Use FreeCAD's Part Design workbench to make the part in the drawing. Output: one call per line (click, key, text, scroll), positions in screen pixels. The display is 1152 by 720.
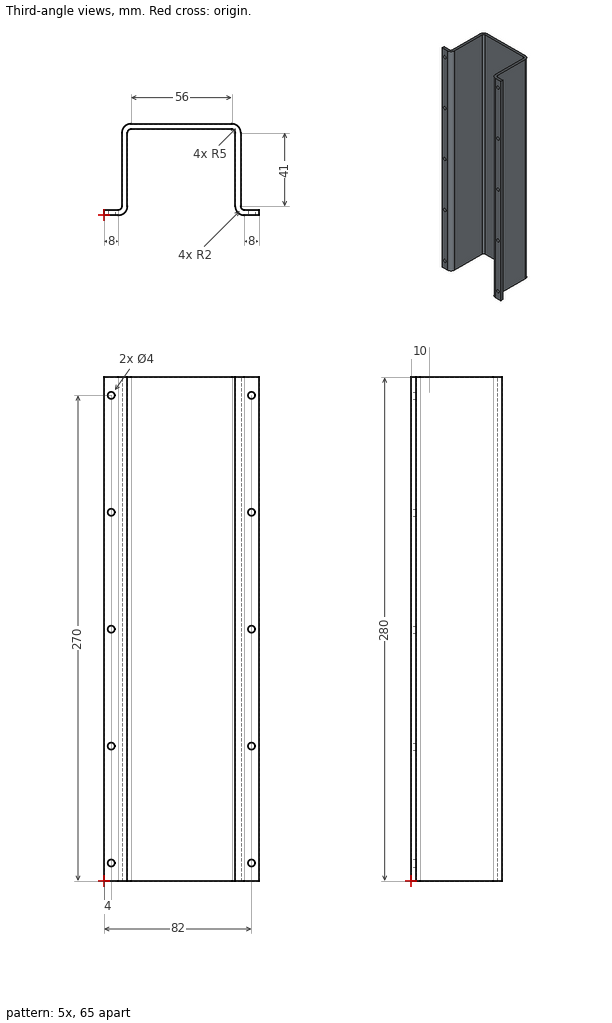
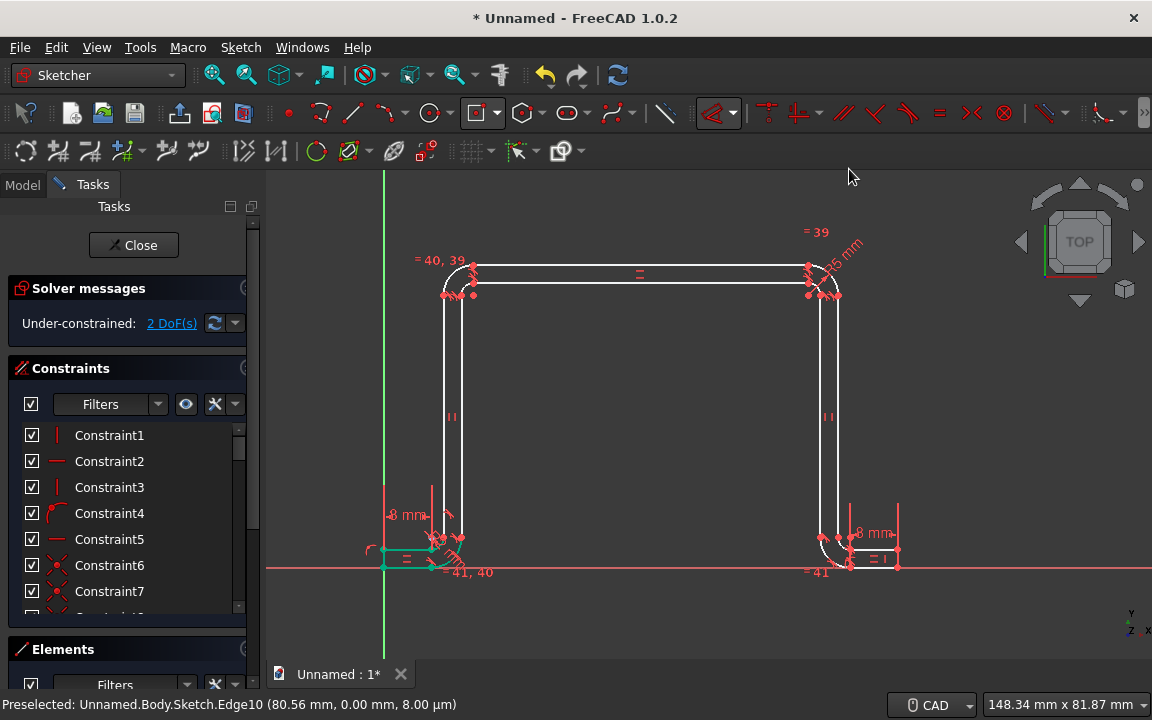
click(838, 465)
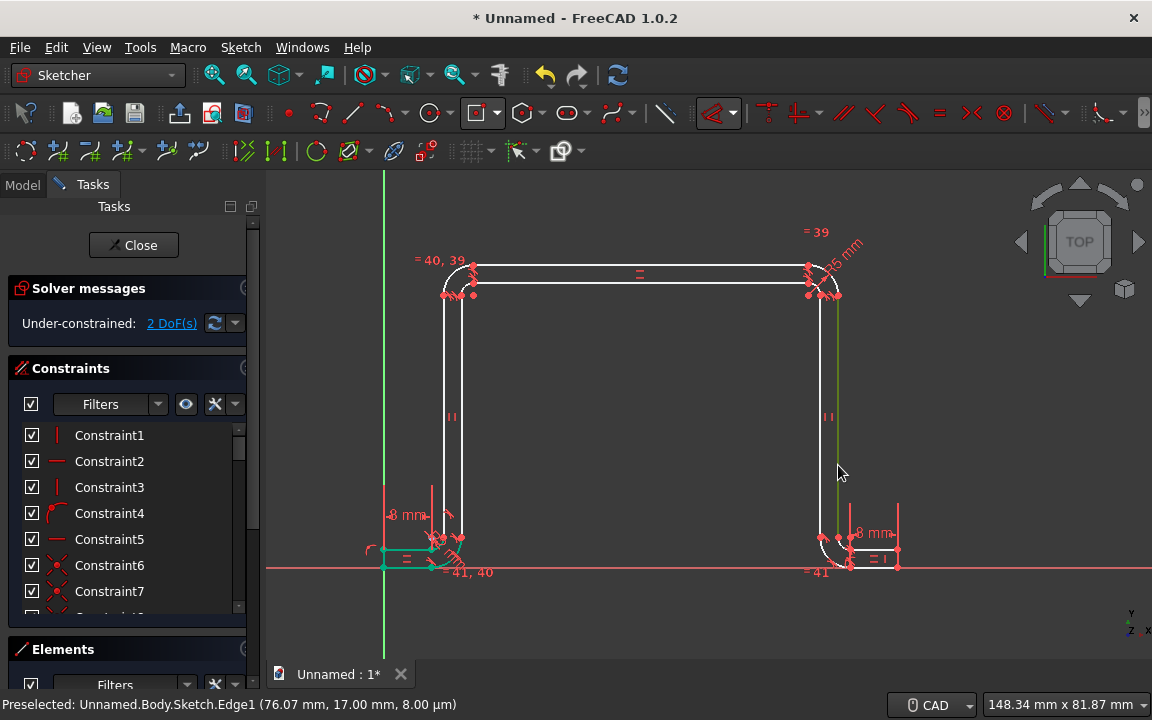
key(i)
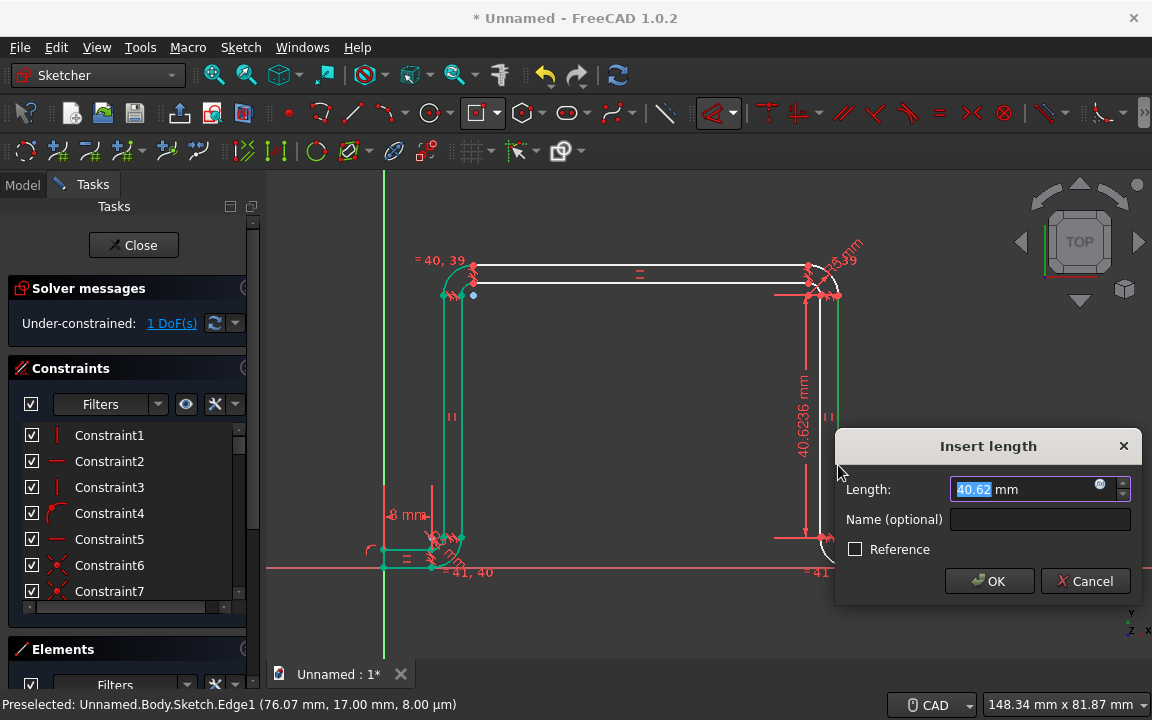
text(41)
key(Return)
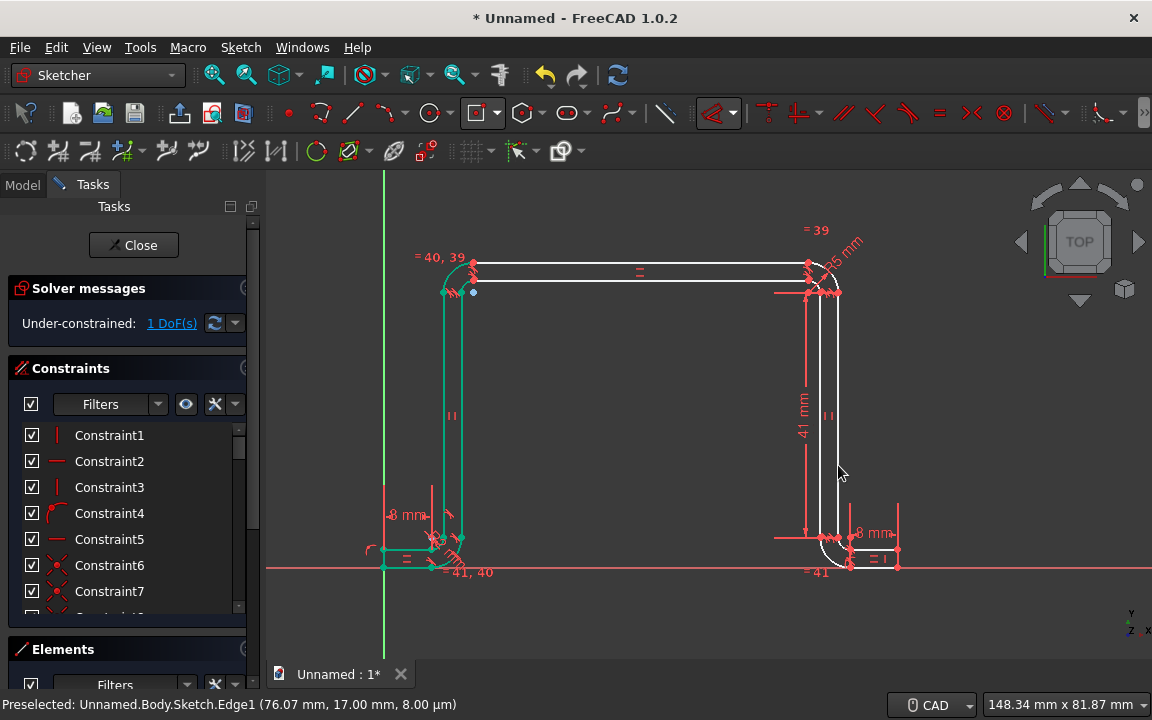
click(708, 263)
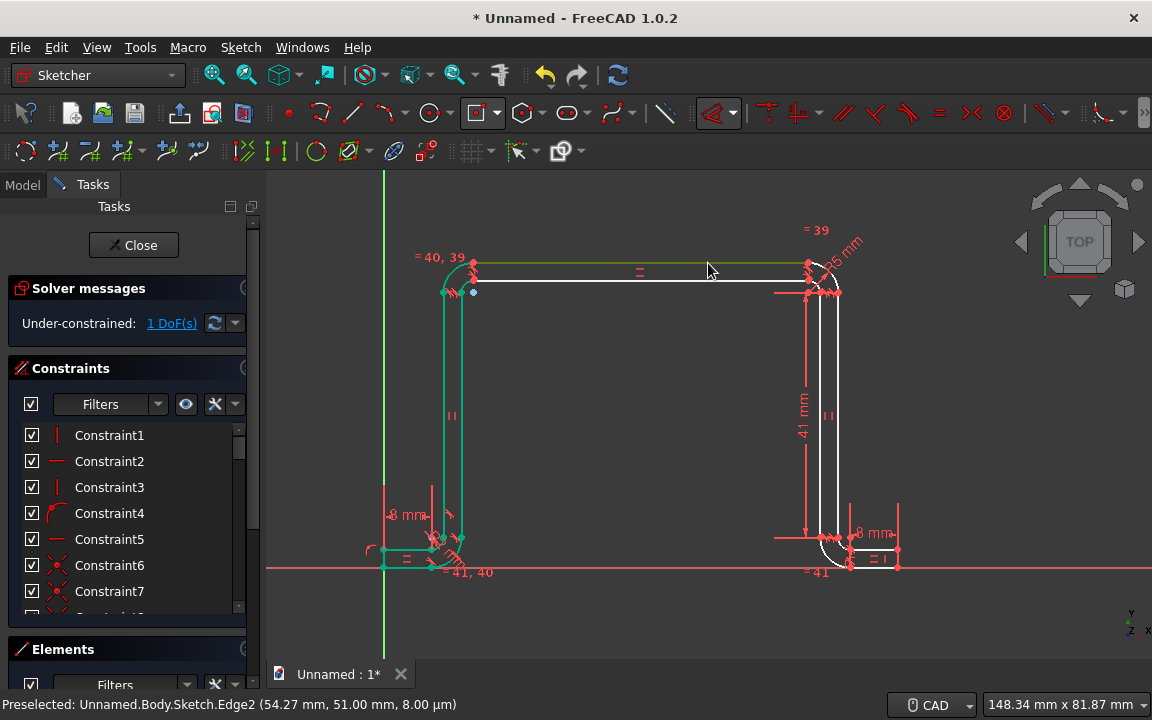
click(736, 114)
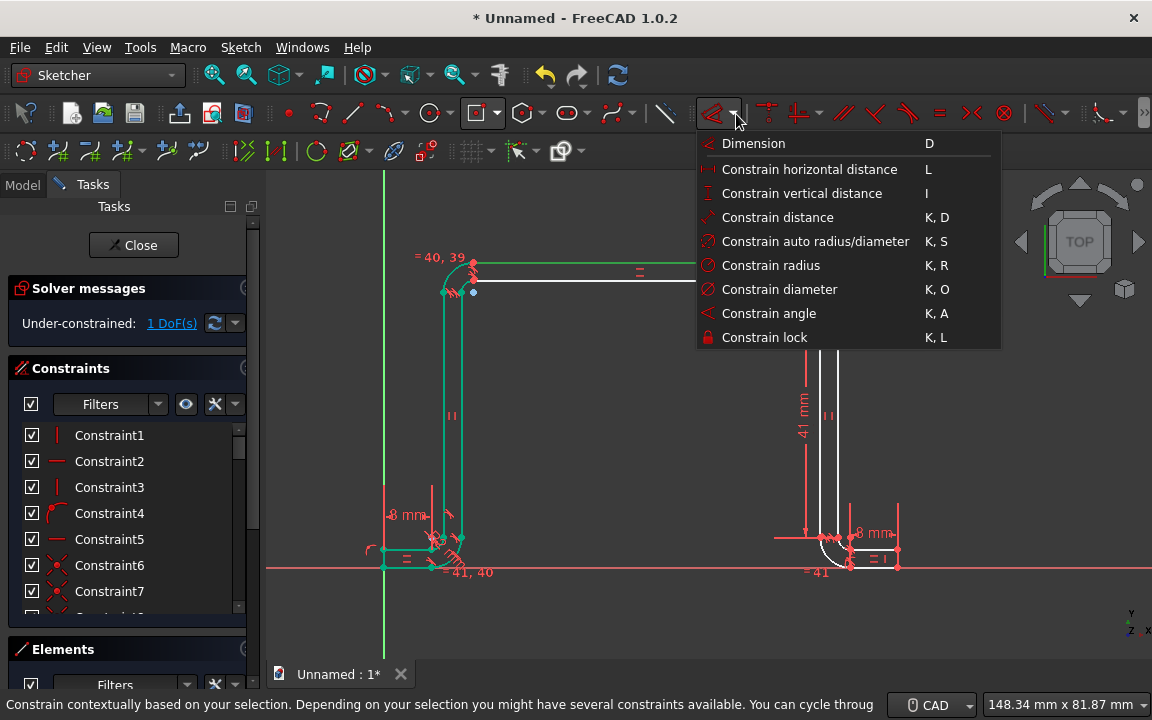
click(849, 169)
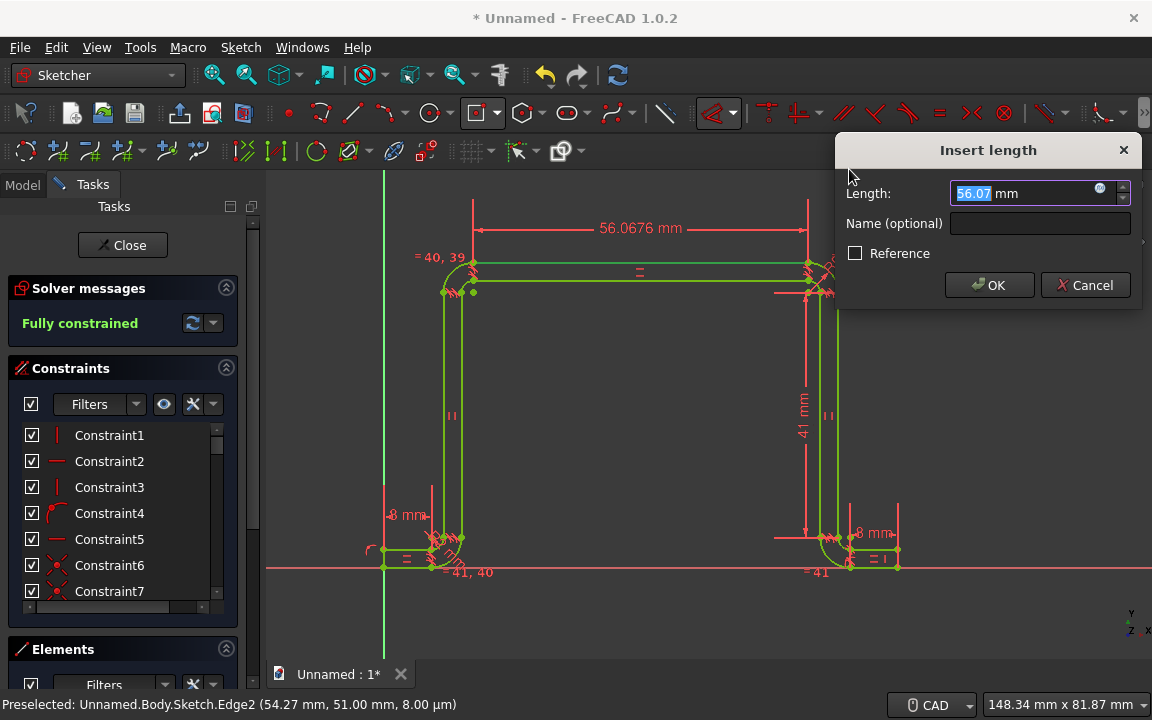
text(56)
key(Return)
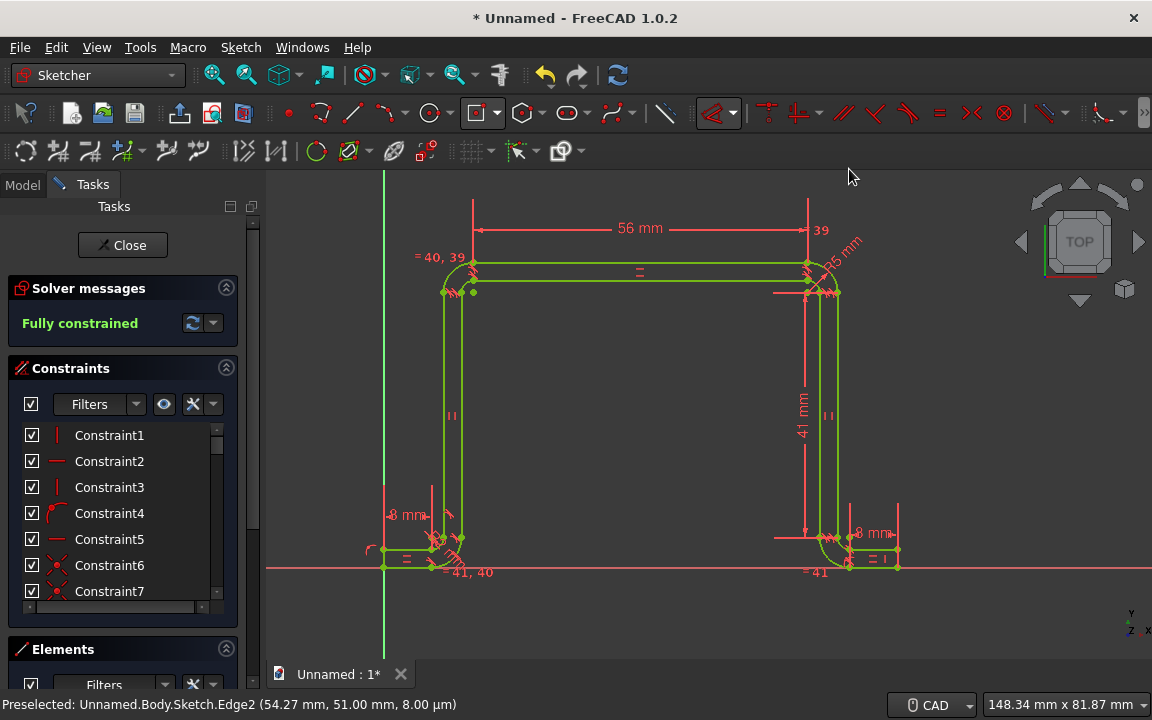
click(123, 245)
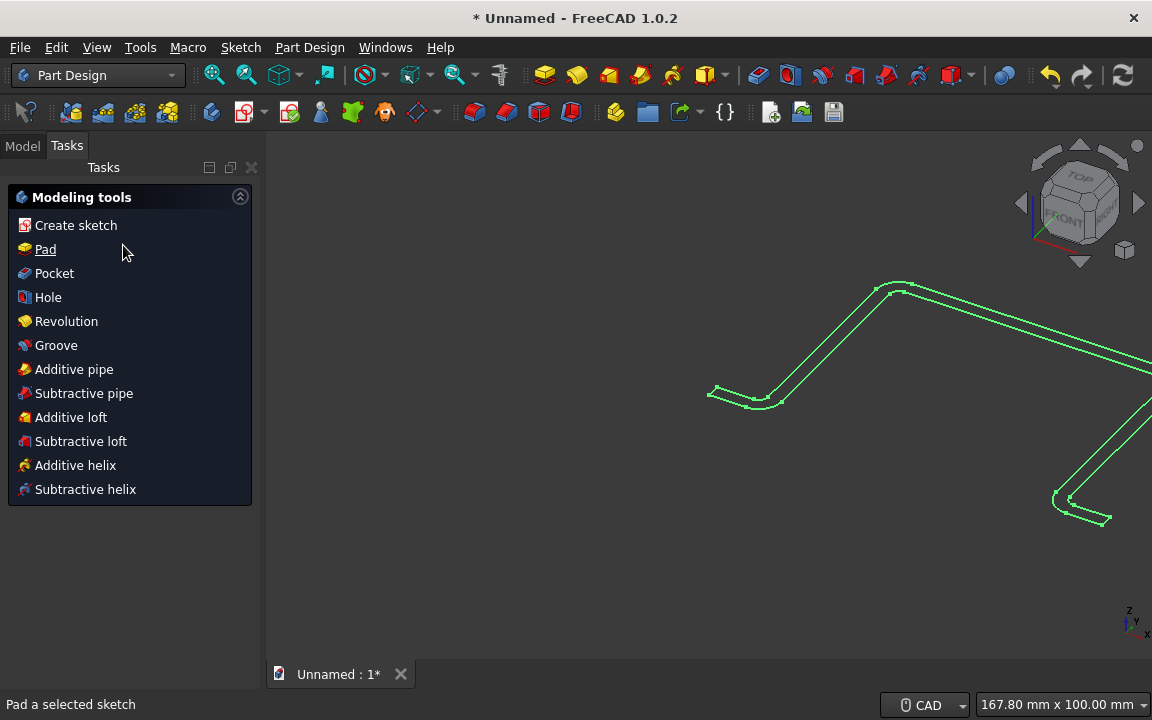
click(546, 76)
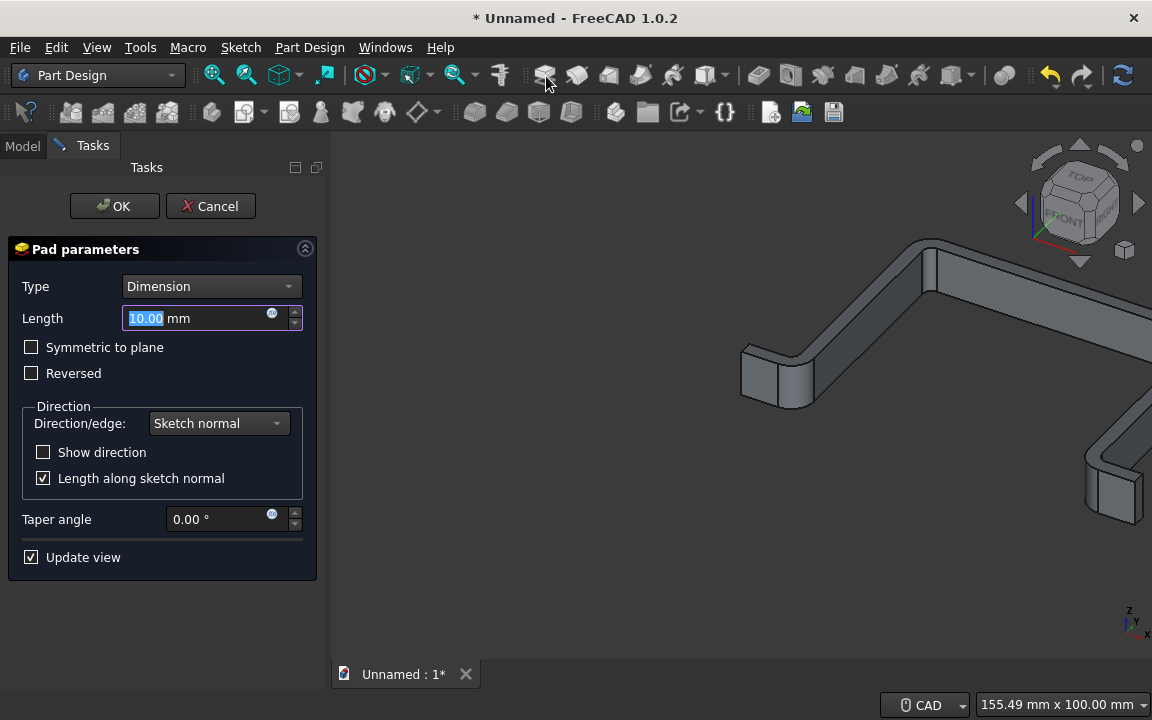
text(280)
key(Tab)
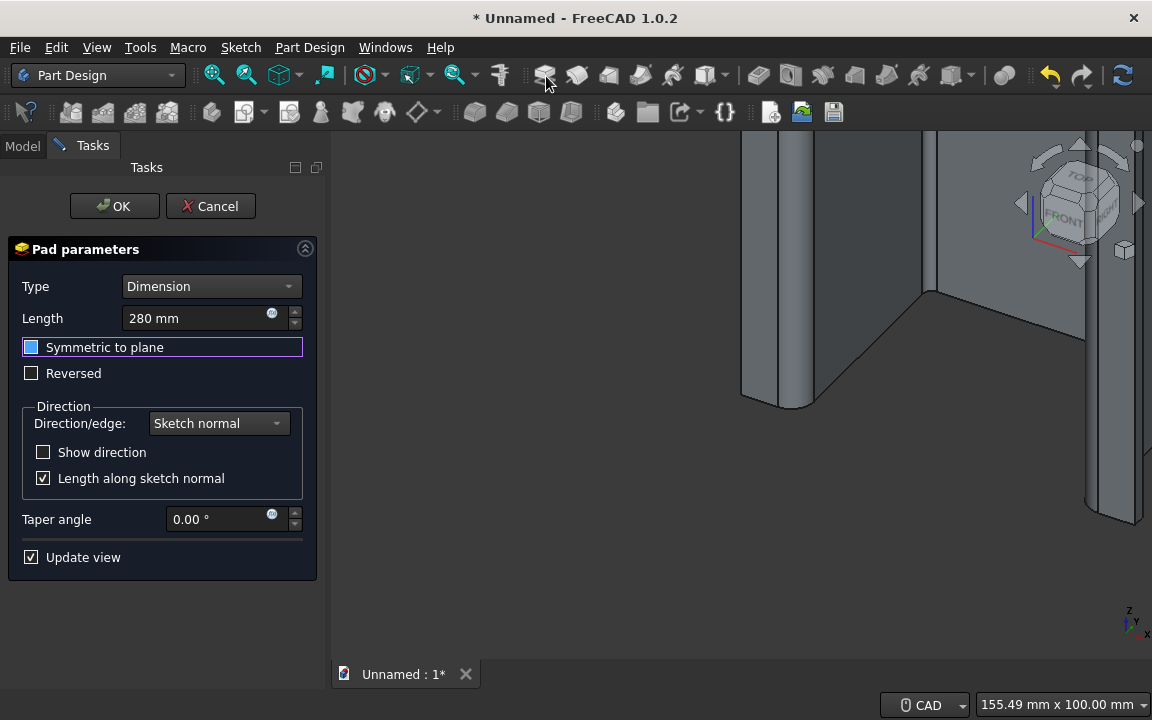
click(115, 206)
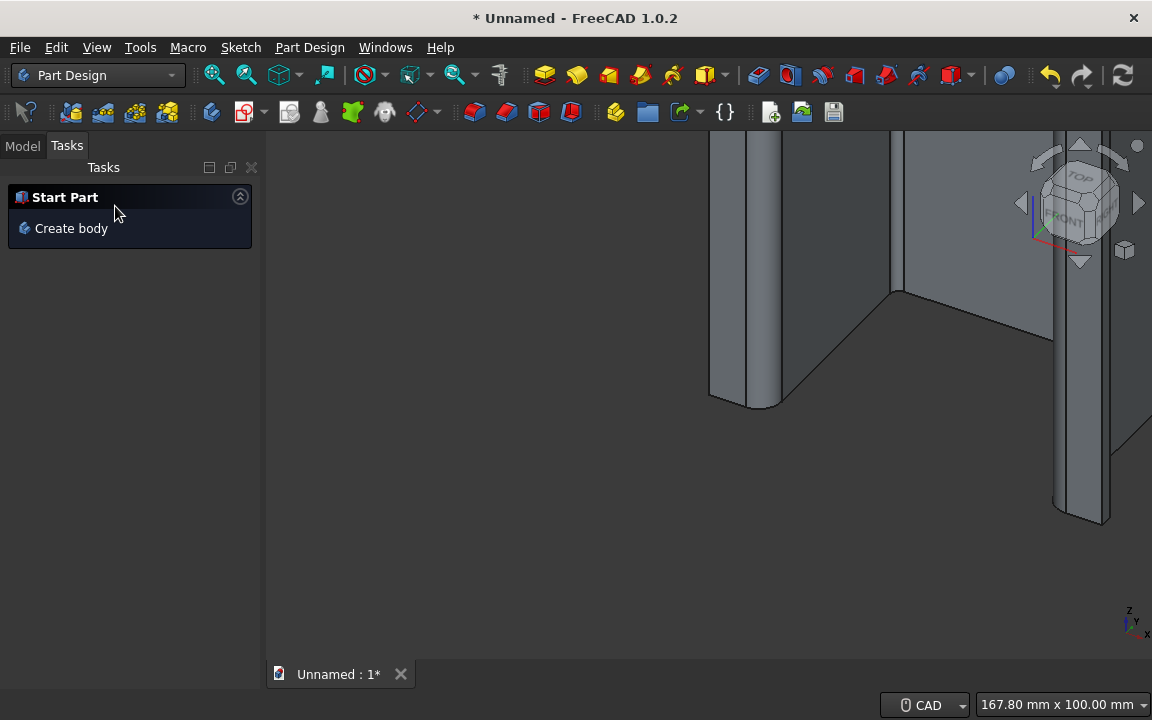
click(216, 76)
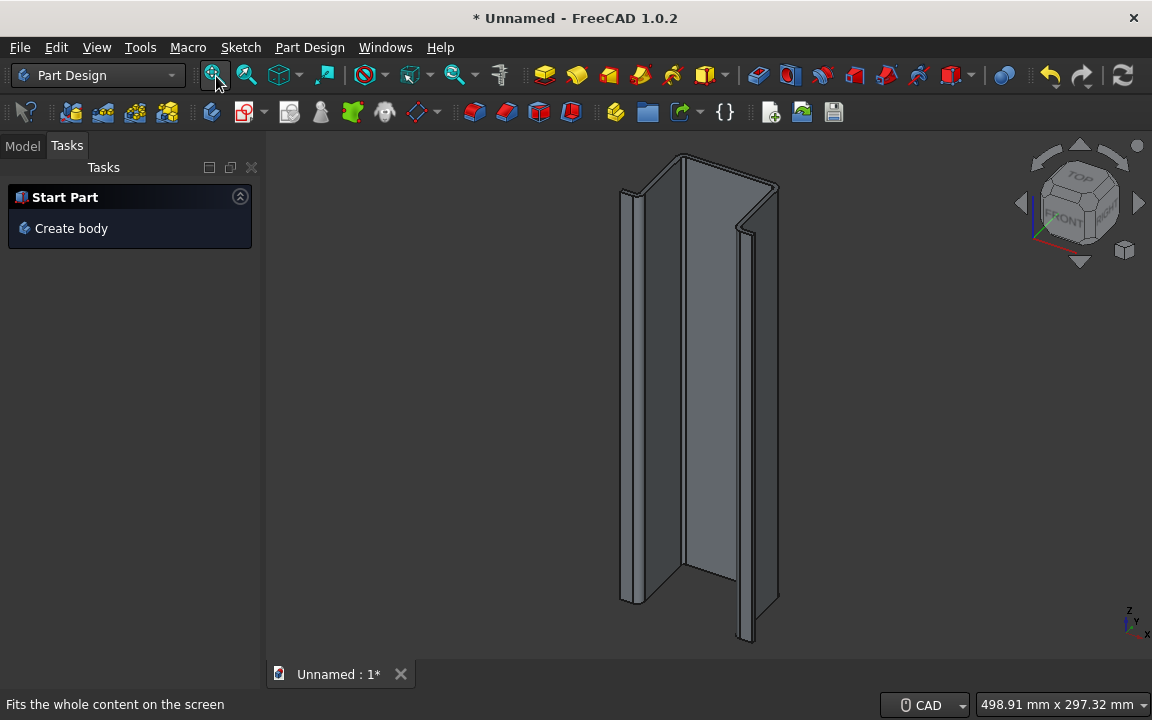
key(0)